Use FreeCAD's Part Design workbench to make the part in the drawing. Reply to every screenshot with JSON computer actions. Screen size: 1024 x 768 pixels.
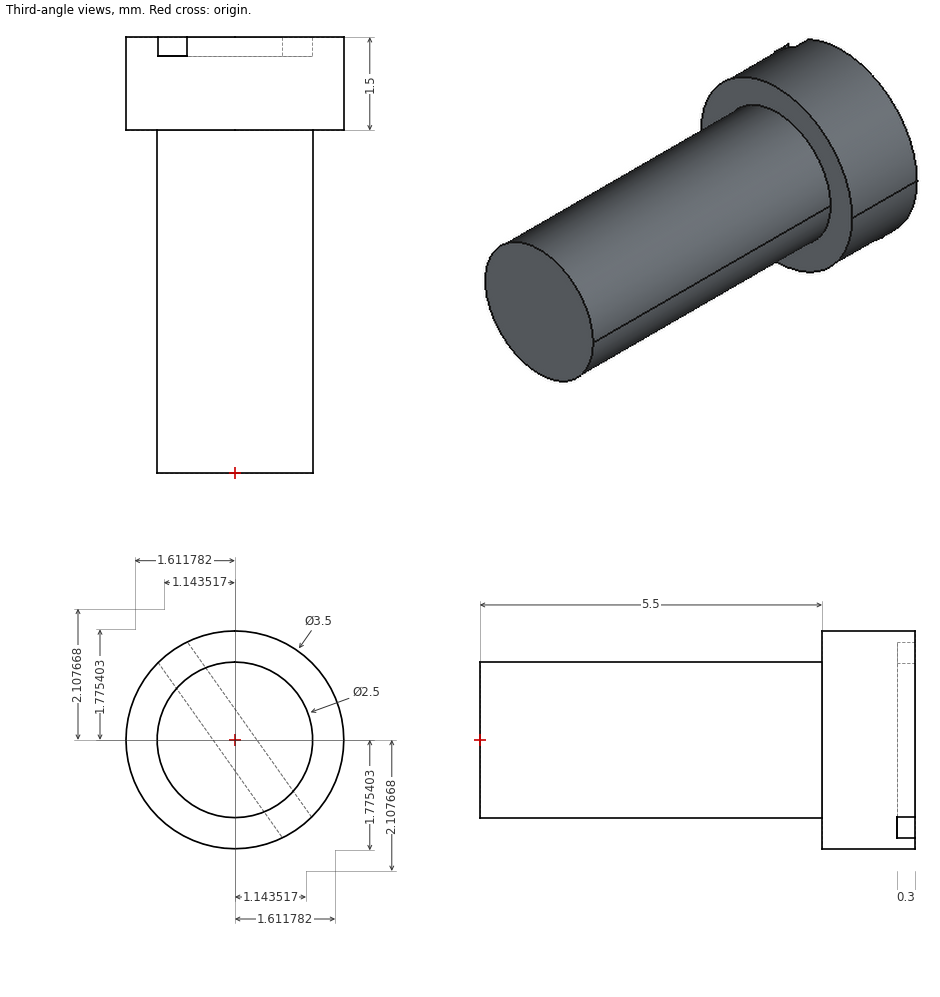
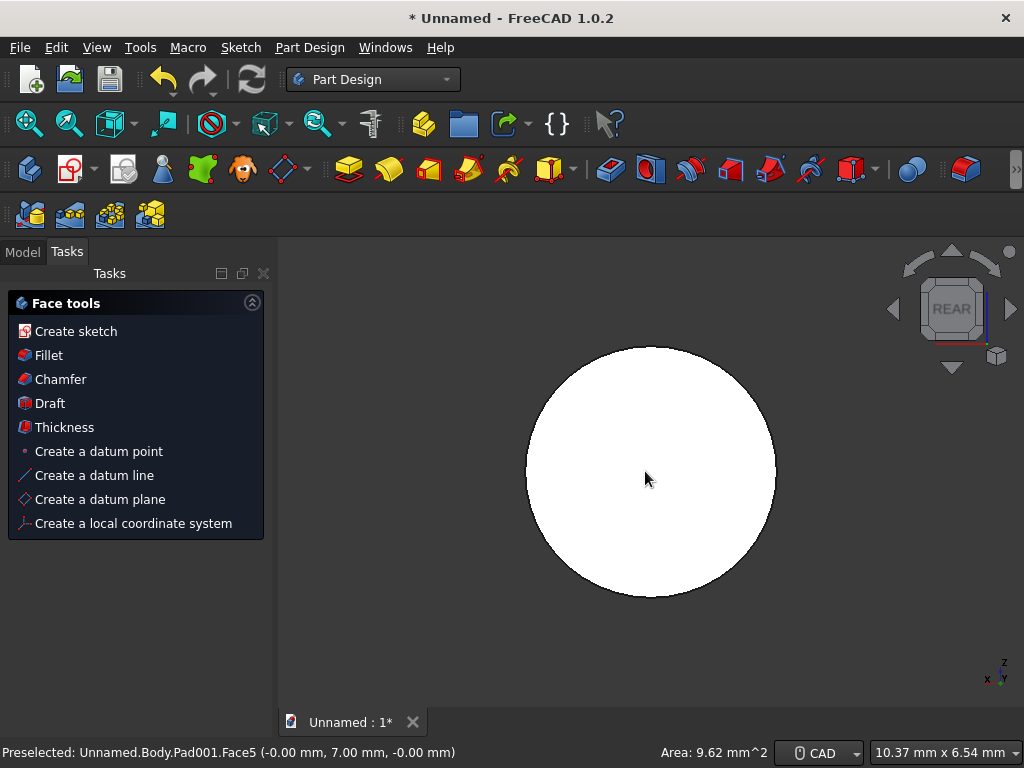
{"action": "left_click", "coordinate": [70, 170]}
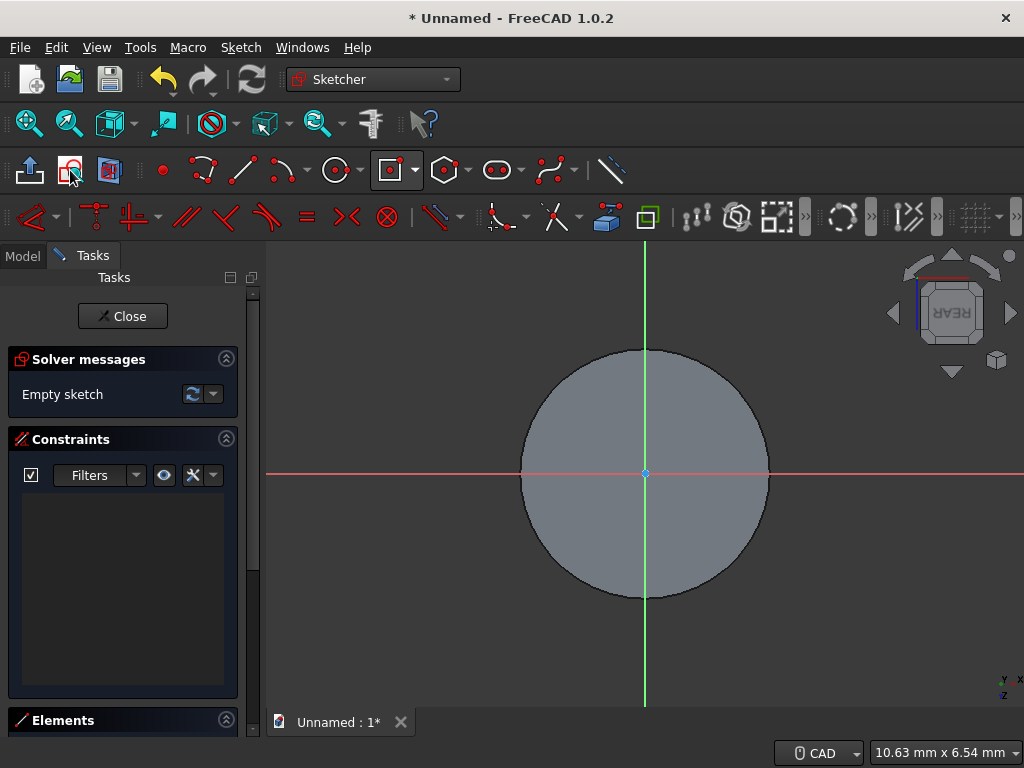
{"action": "key", "text": "g m"}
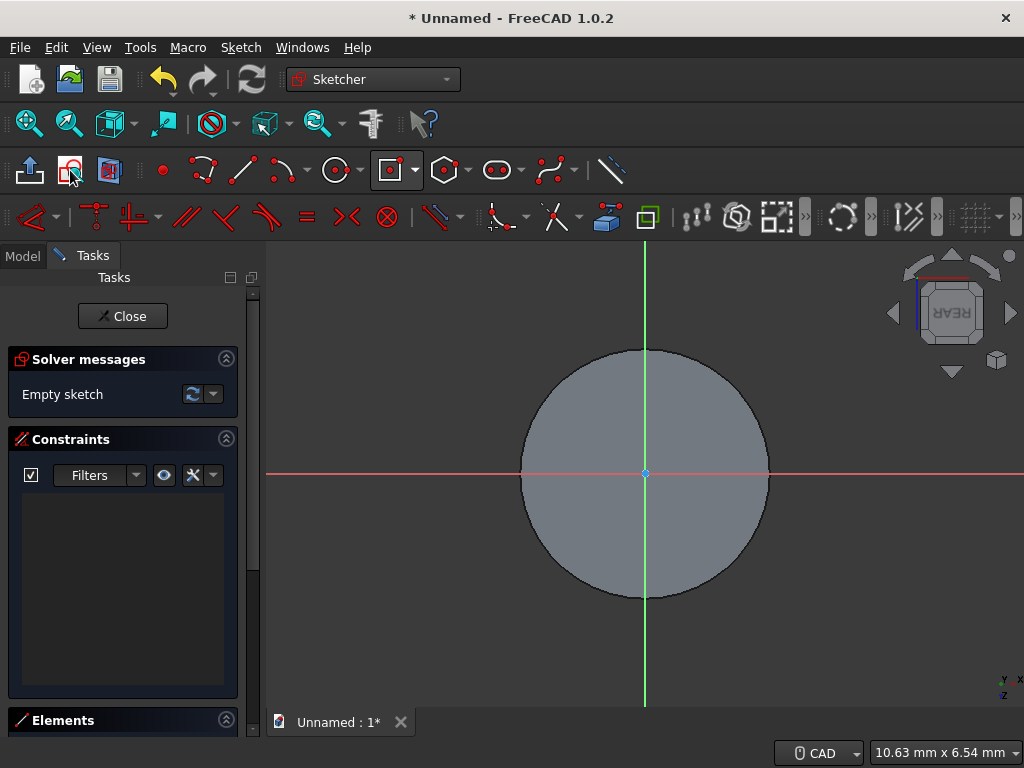
{"action": "left_click", "coordinate": [530, 601]}
{"action": "left_click", "coordinate": [563, 624]}
{"action": "left_click", "coordinate": [760, 347]}
{"action": "left_click", "coordinate": [727, 324]}
{"action": "left_click", "coordinate": [530, 602]}
{"action": "key", "text": "Escape"}
{"action": "key", "text": "Escape"}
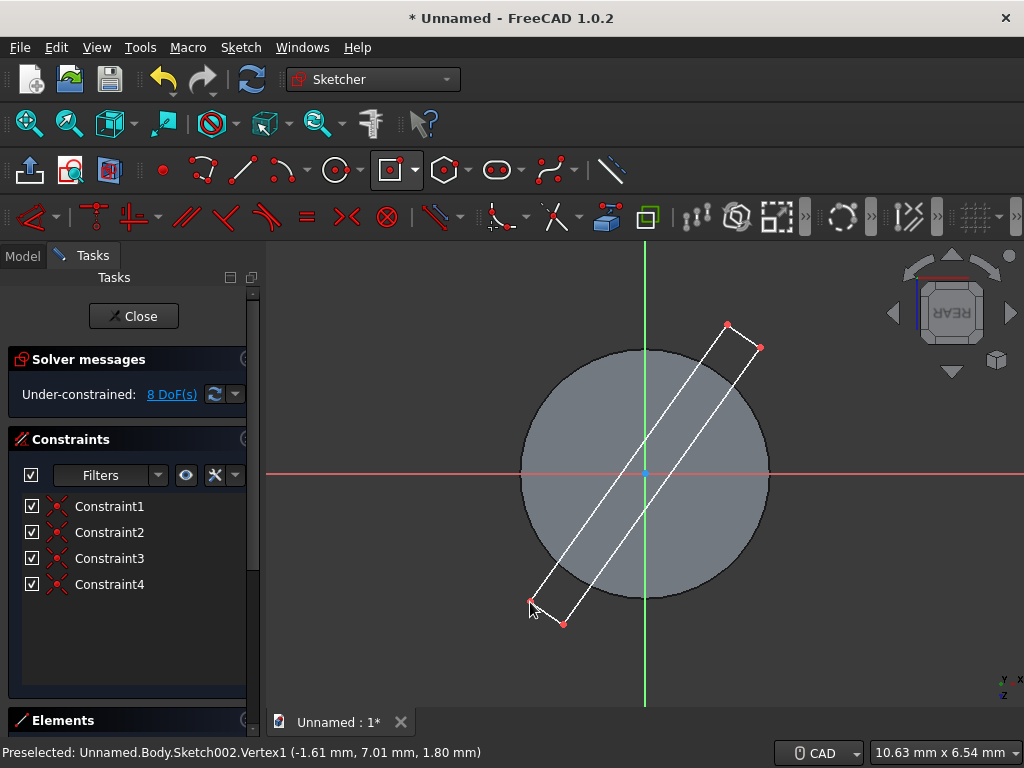
{"action": "key", "text": "d"}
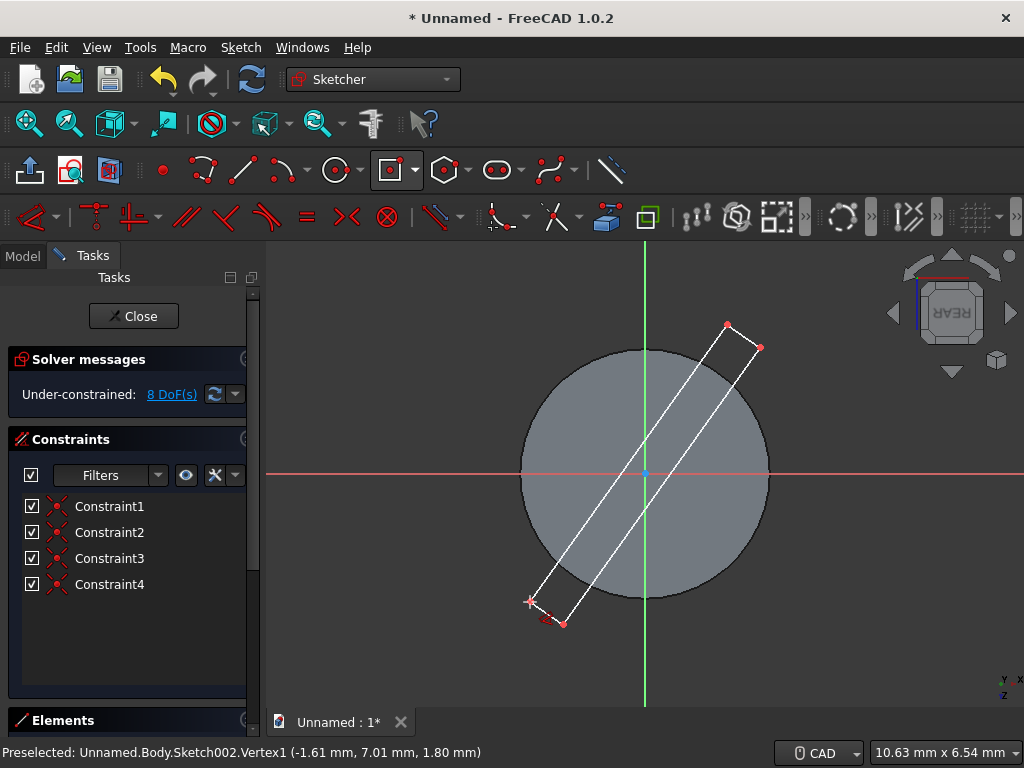
{"action": "left_click", "coordinate": [530, 602]}
{"action": "left_click", "coordinate": [587, 636]}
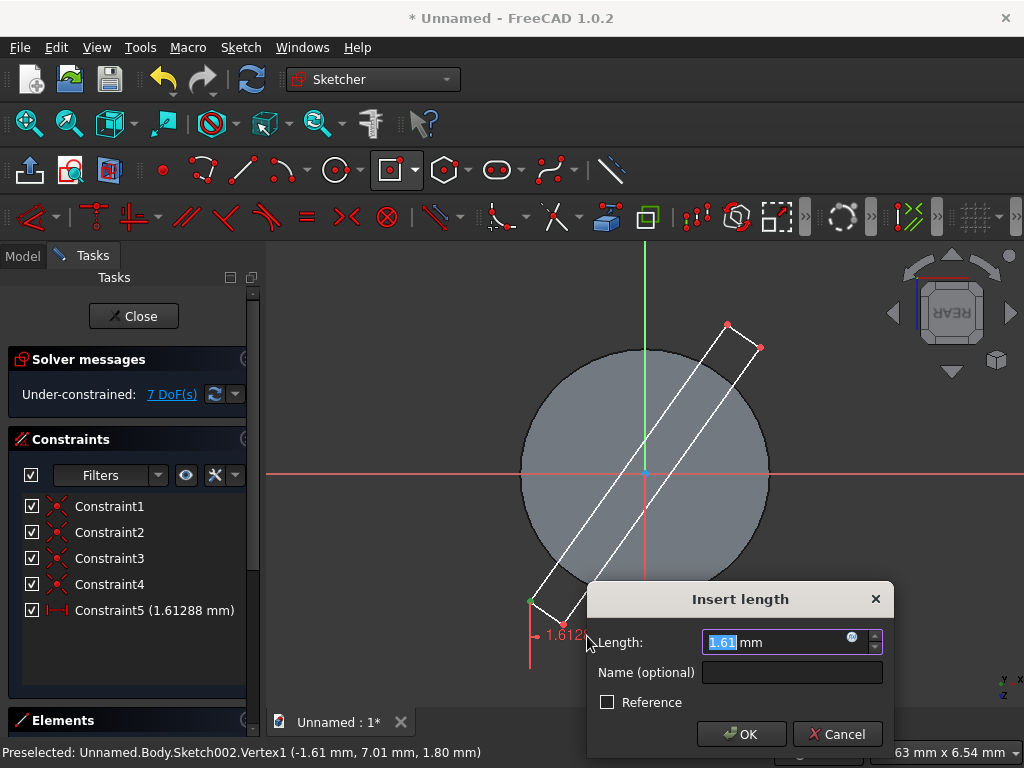
{"action": "type", "text": "1.611782"}
{"action": "key", "text": "Return"}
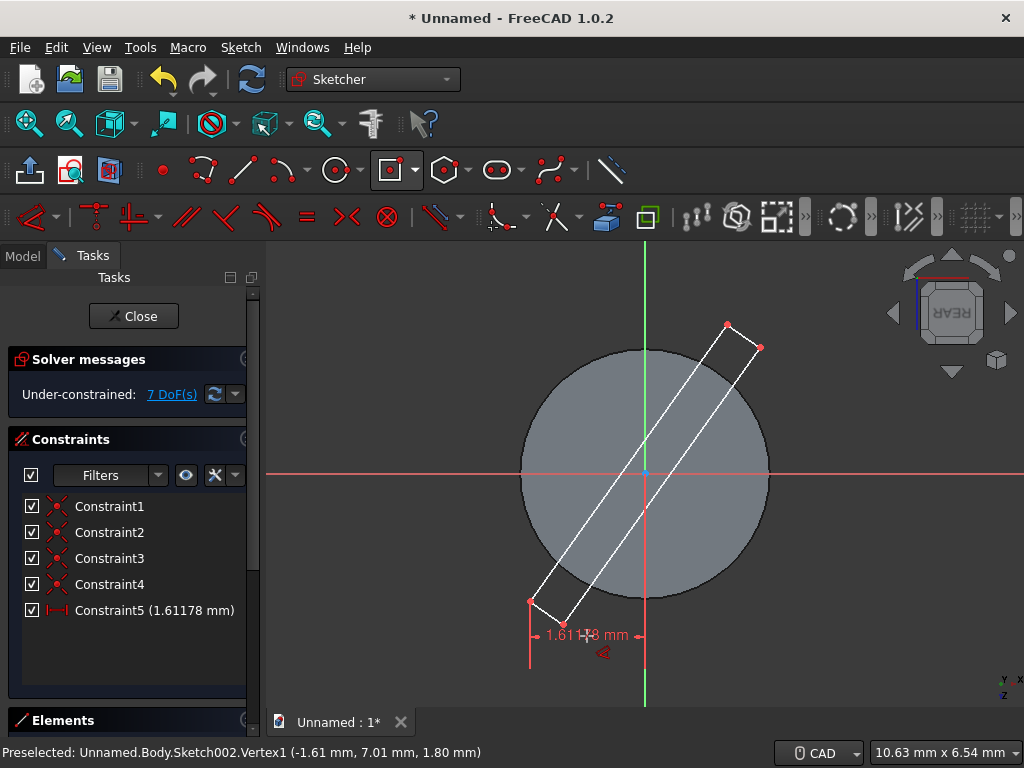
{"action": "left_click", "coordinate": [530, 602]}
{"action": "left_click", "coordinate": [496, 538]}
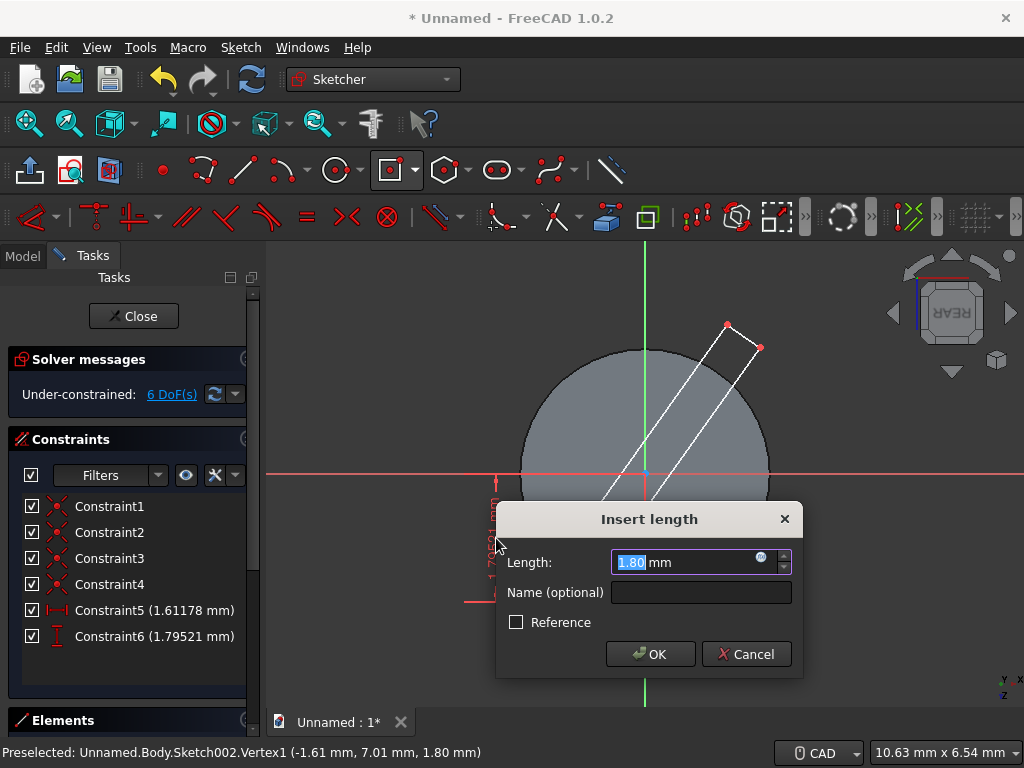
{"action": "type", "text": "1.775403"}
{"action": "key", "text": "Return"}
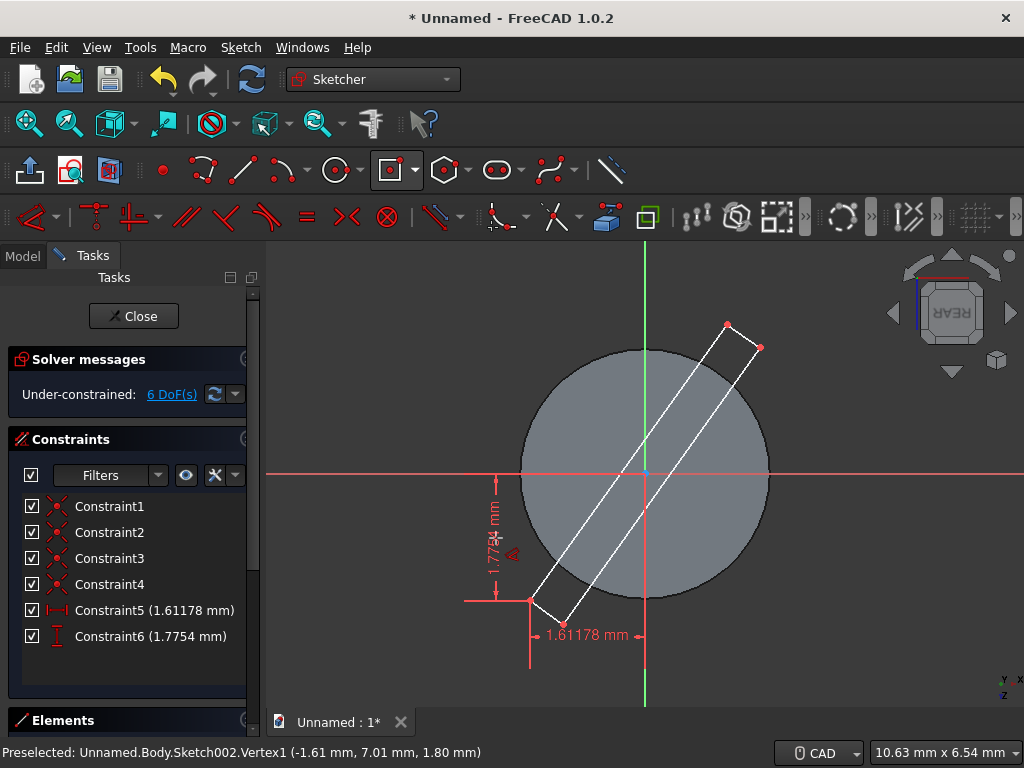
{"action": "left_click", "coordinate": [563, 625]}
{"action": "left_click", "coordinate": [604, 659]}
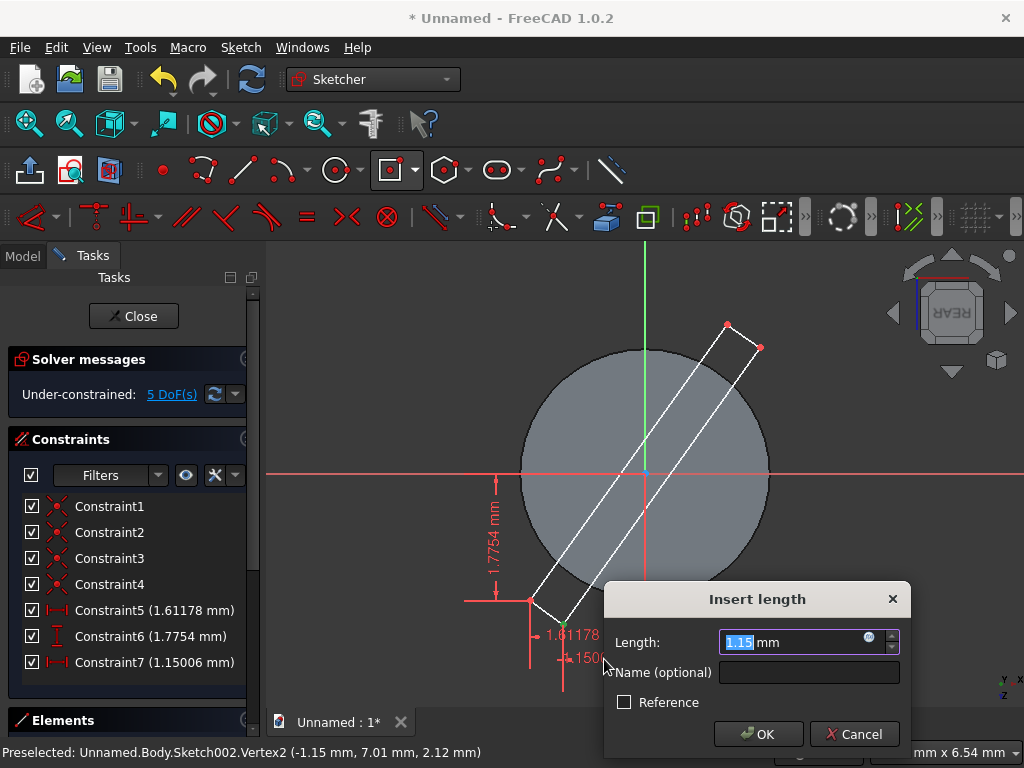
{"action": "type", "text": "1.143517"}
{"action": "key", "text": "Return"}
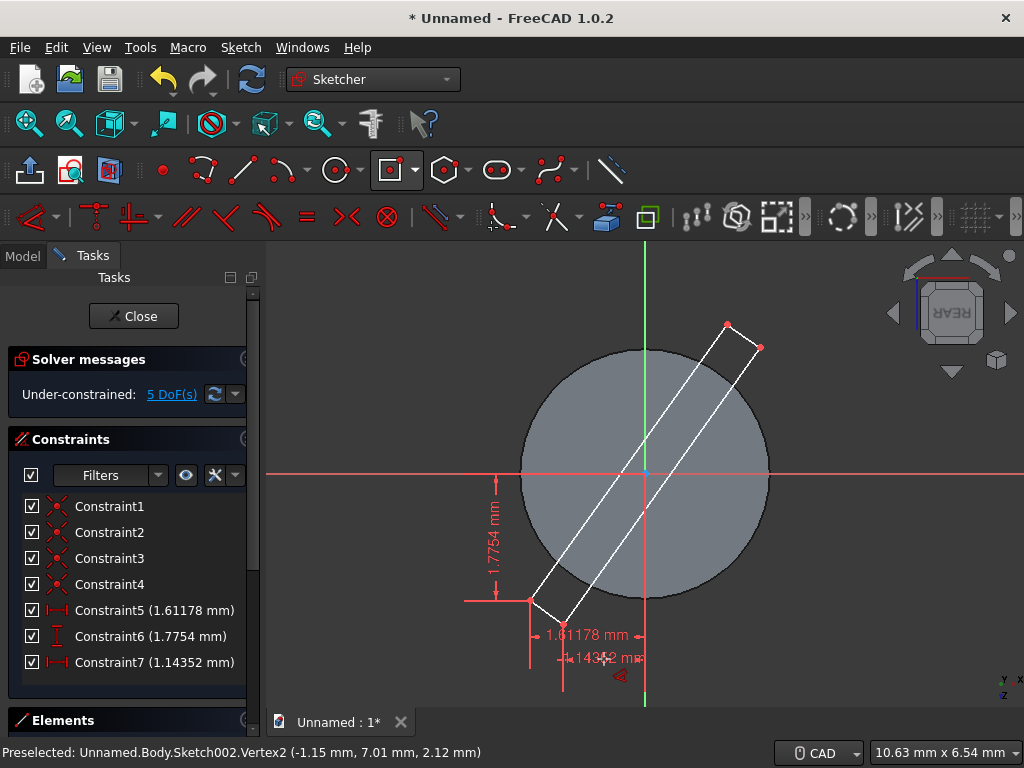
{"action": "left_click", "coordinate": [563, 625]}
{"action": "left_click", "coordinate": [529, 515]}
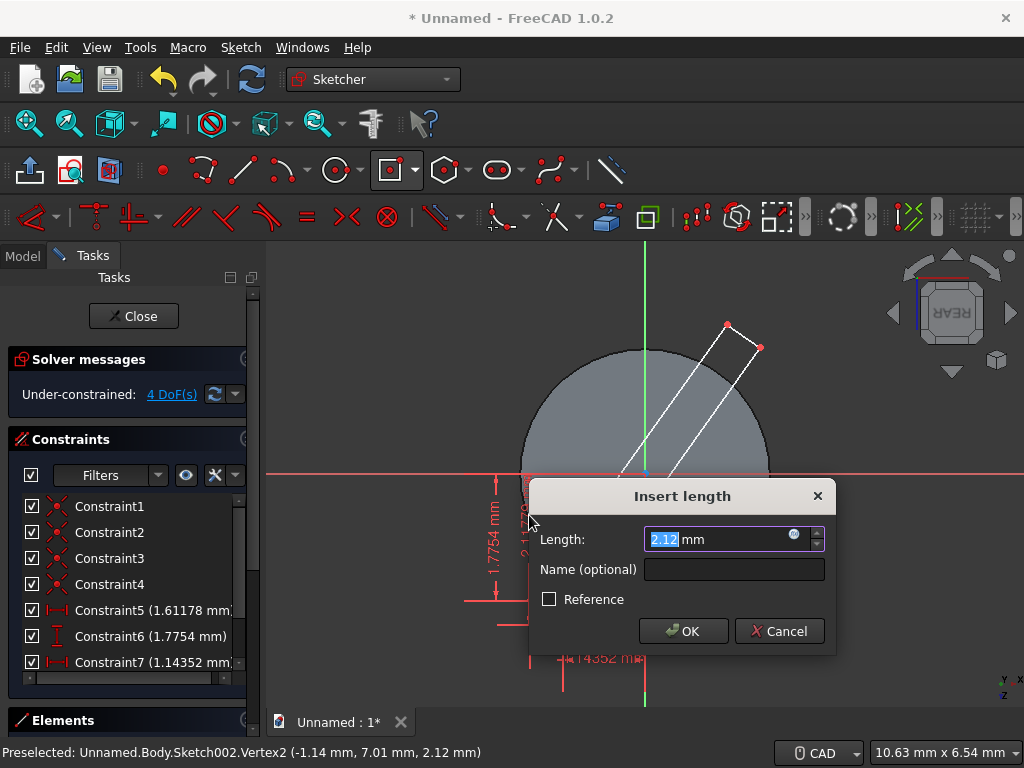
{"action": "type", "text": "2.107668"}
{"action": "key", "text": "Return"}